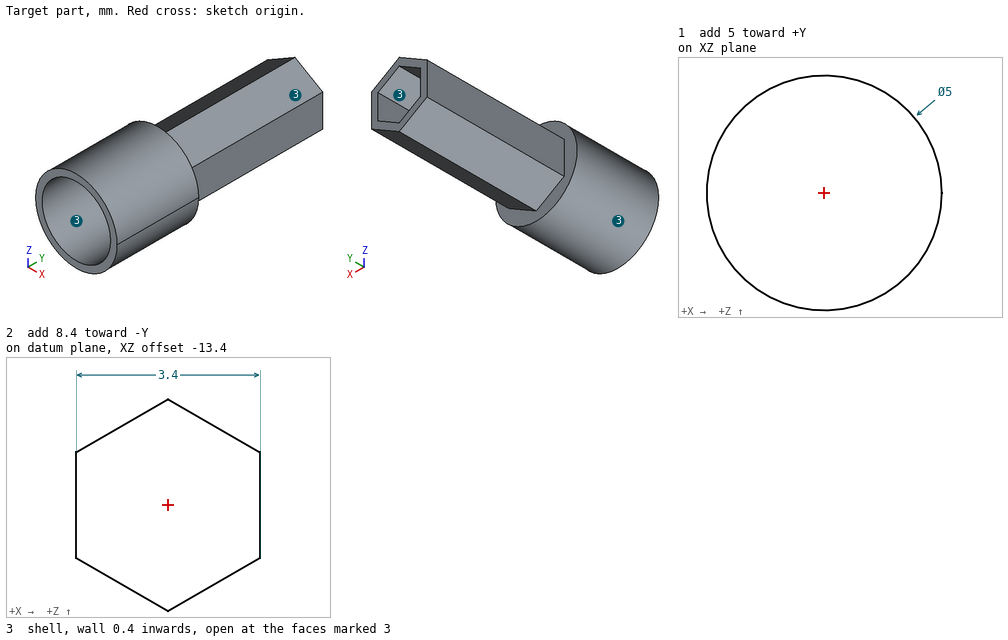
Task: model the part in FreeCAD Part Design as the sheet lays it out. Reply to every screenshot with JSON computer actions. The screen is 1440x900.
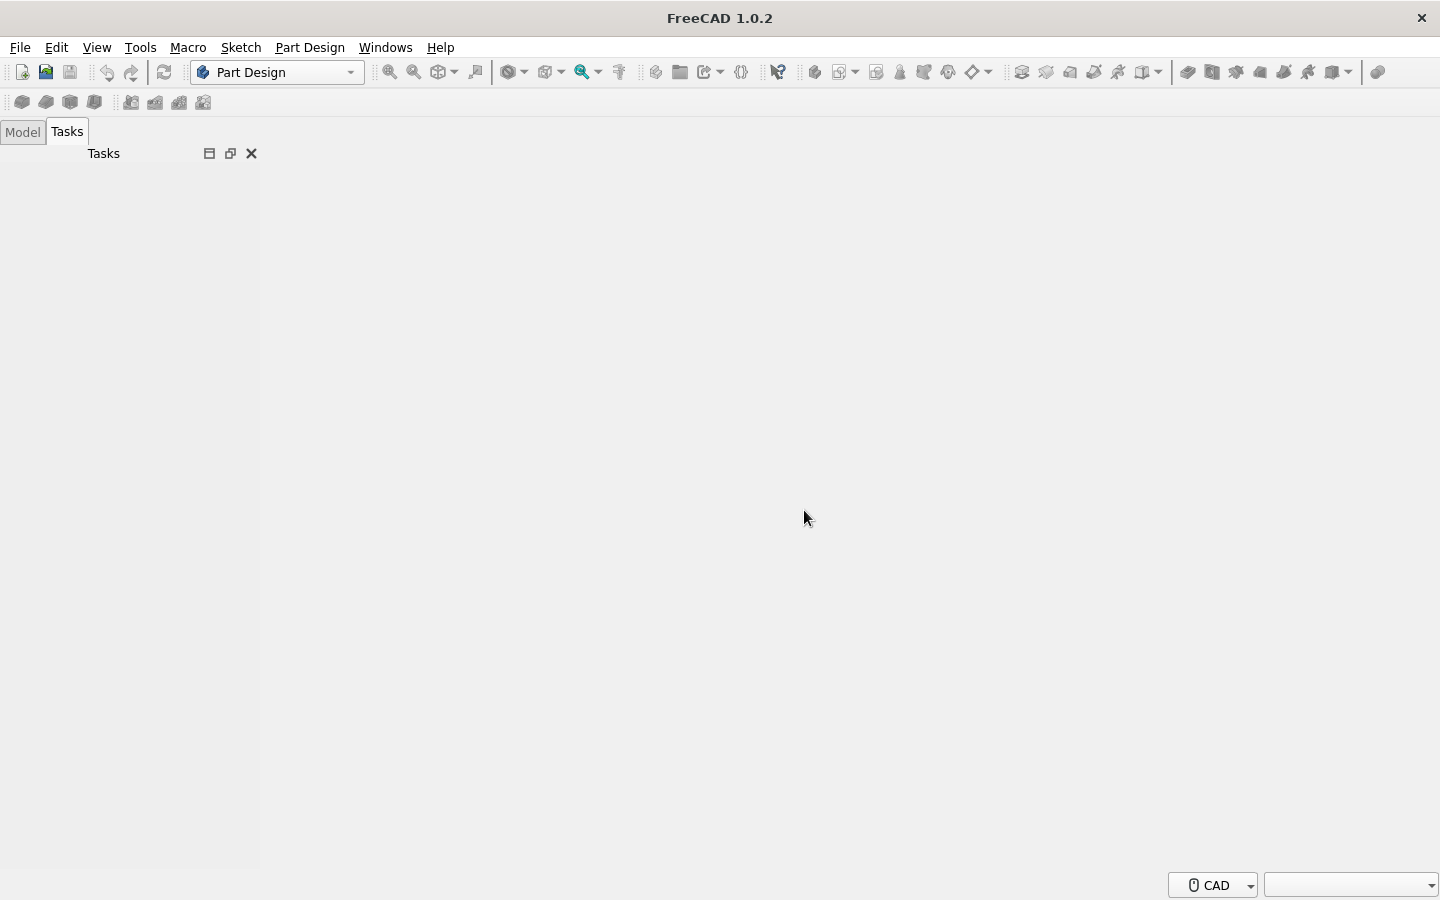
{"action": "left_click", "coordinate": [22, 72]}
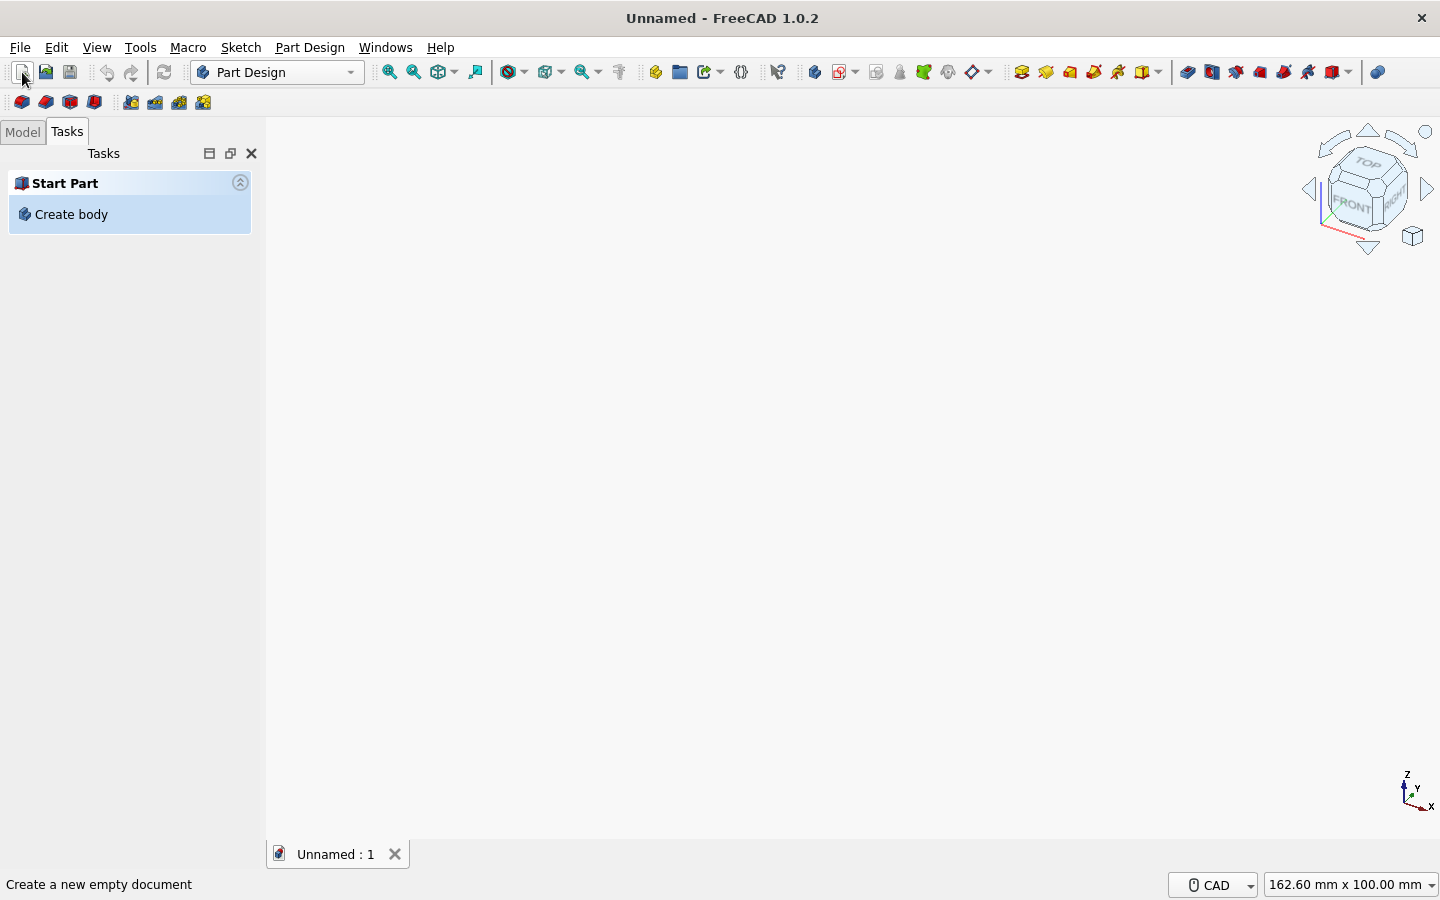
{"action": "left_click", "coordinate": [840, 72]}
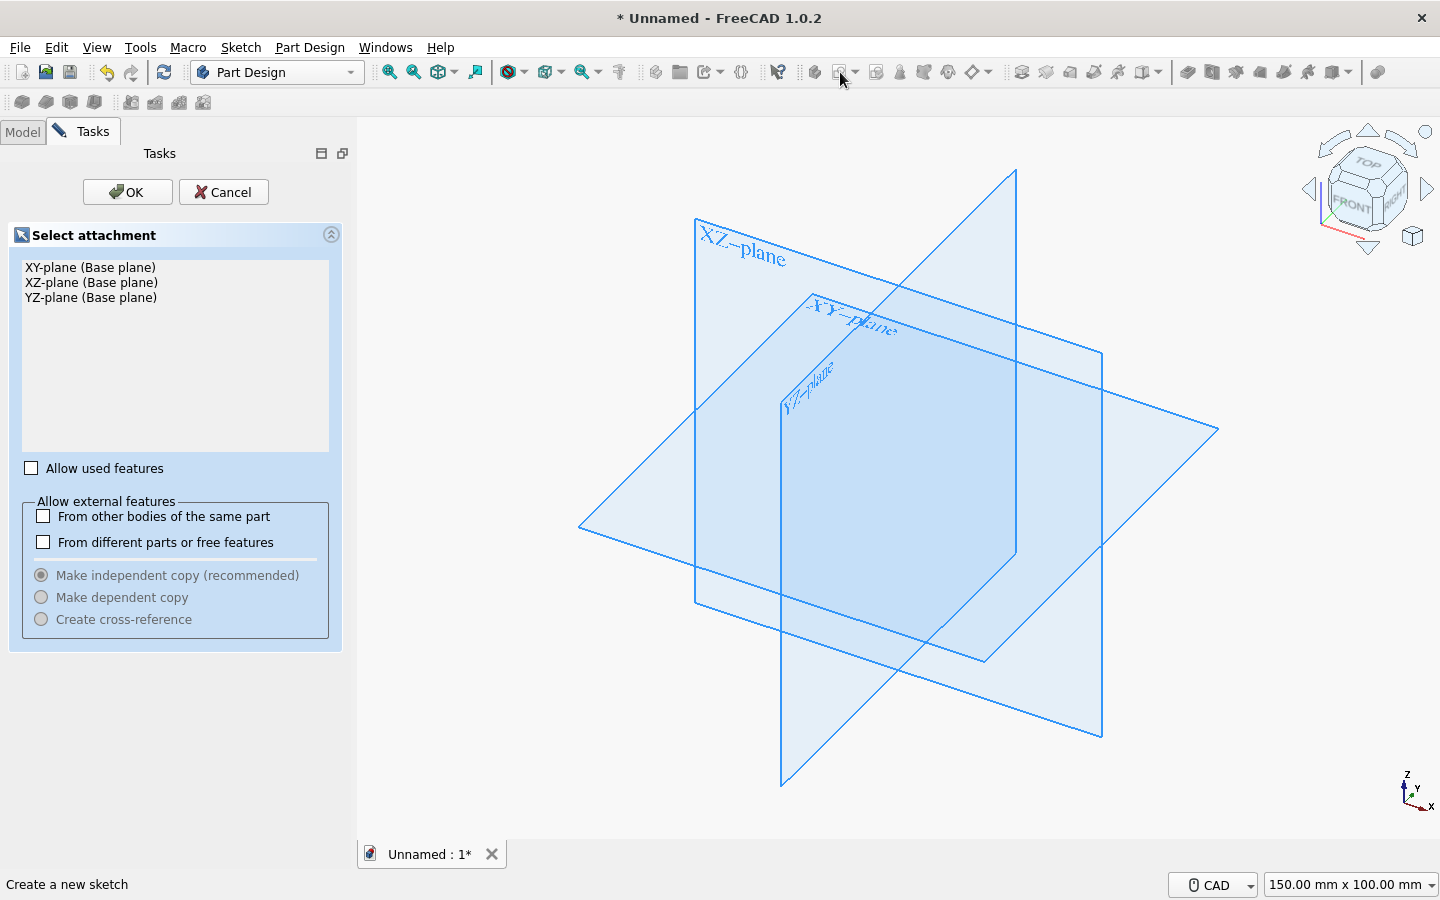
{"action": "left_click", "coordinate": [82, 282]}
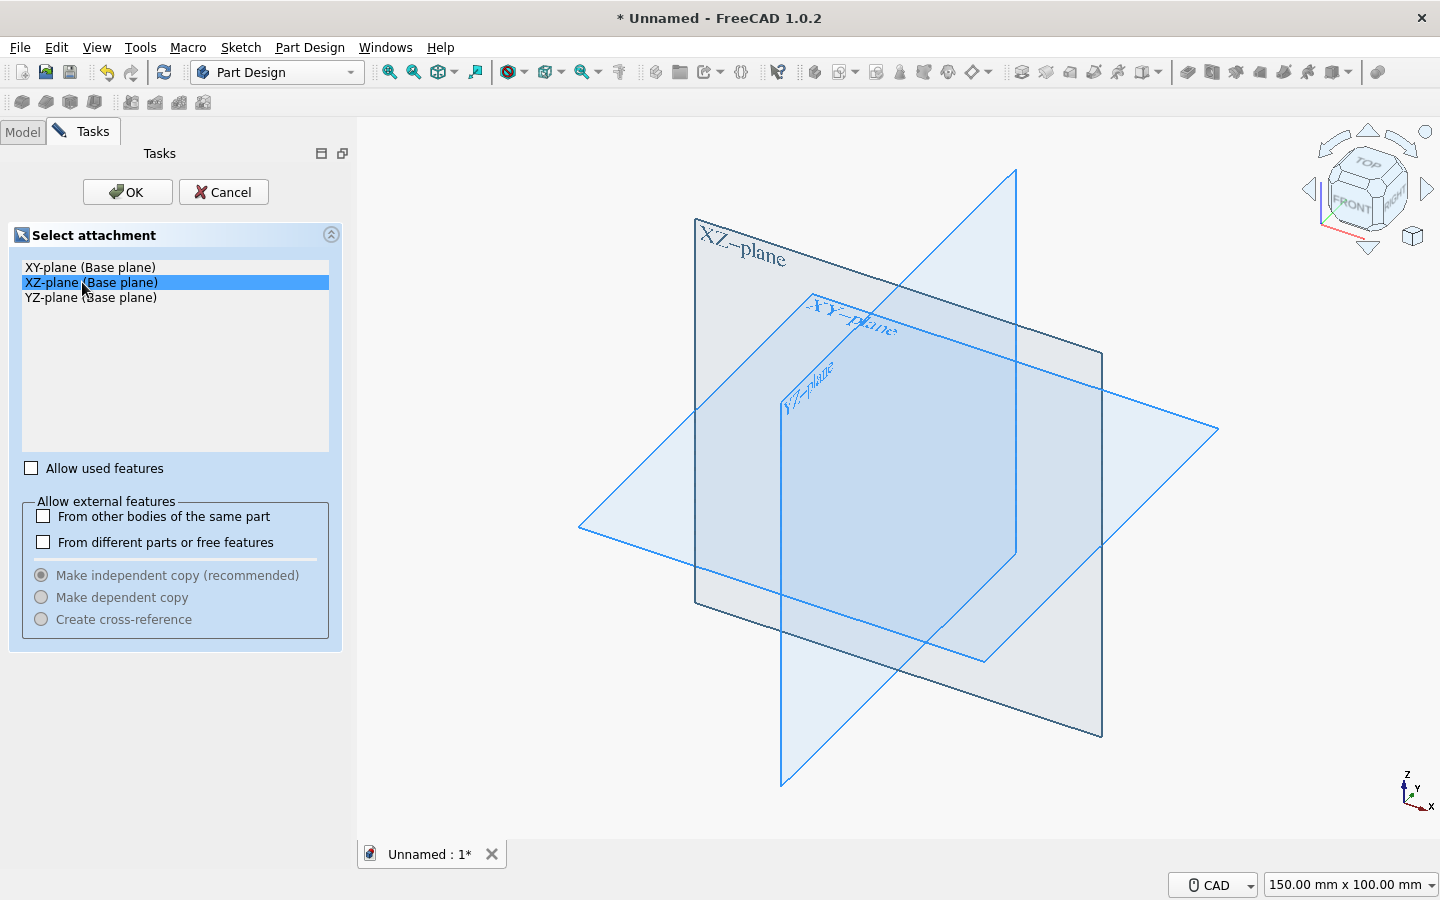
{"action": "left_click", "coordinate": [128, 192]}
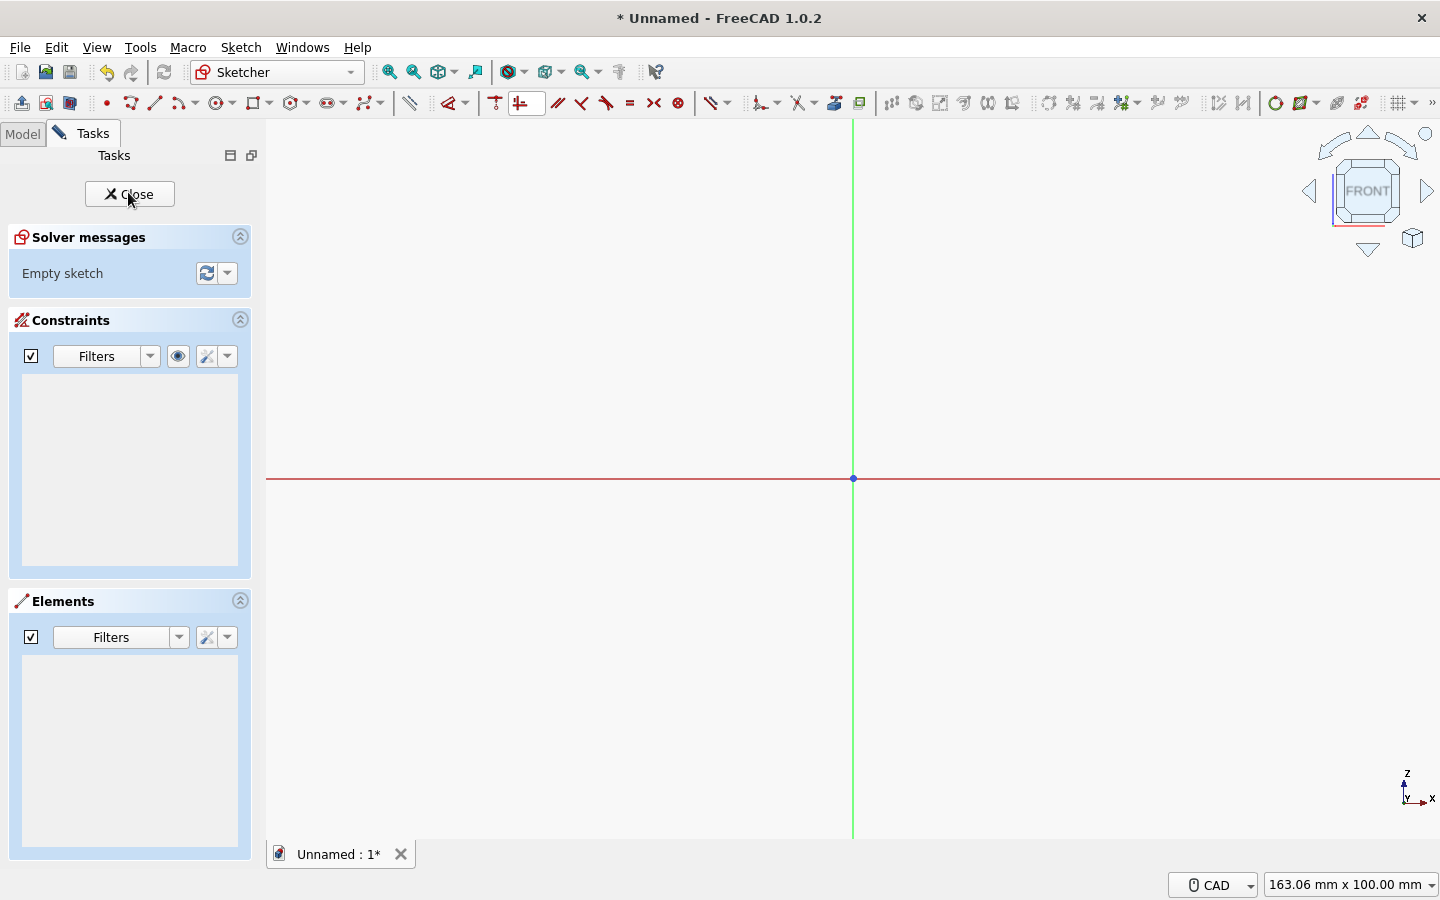
{"action": "scroll", "coordinate": [858, 479], "scroll_direction": "up", "scroll_amount": 13}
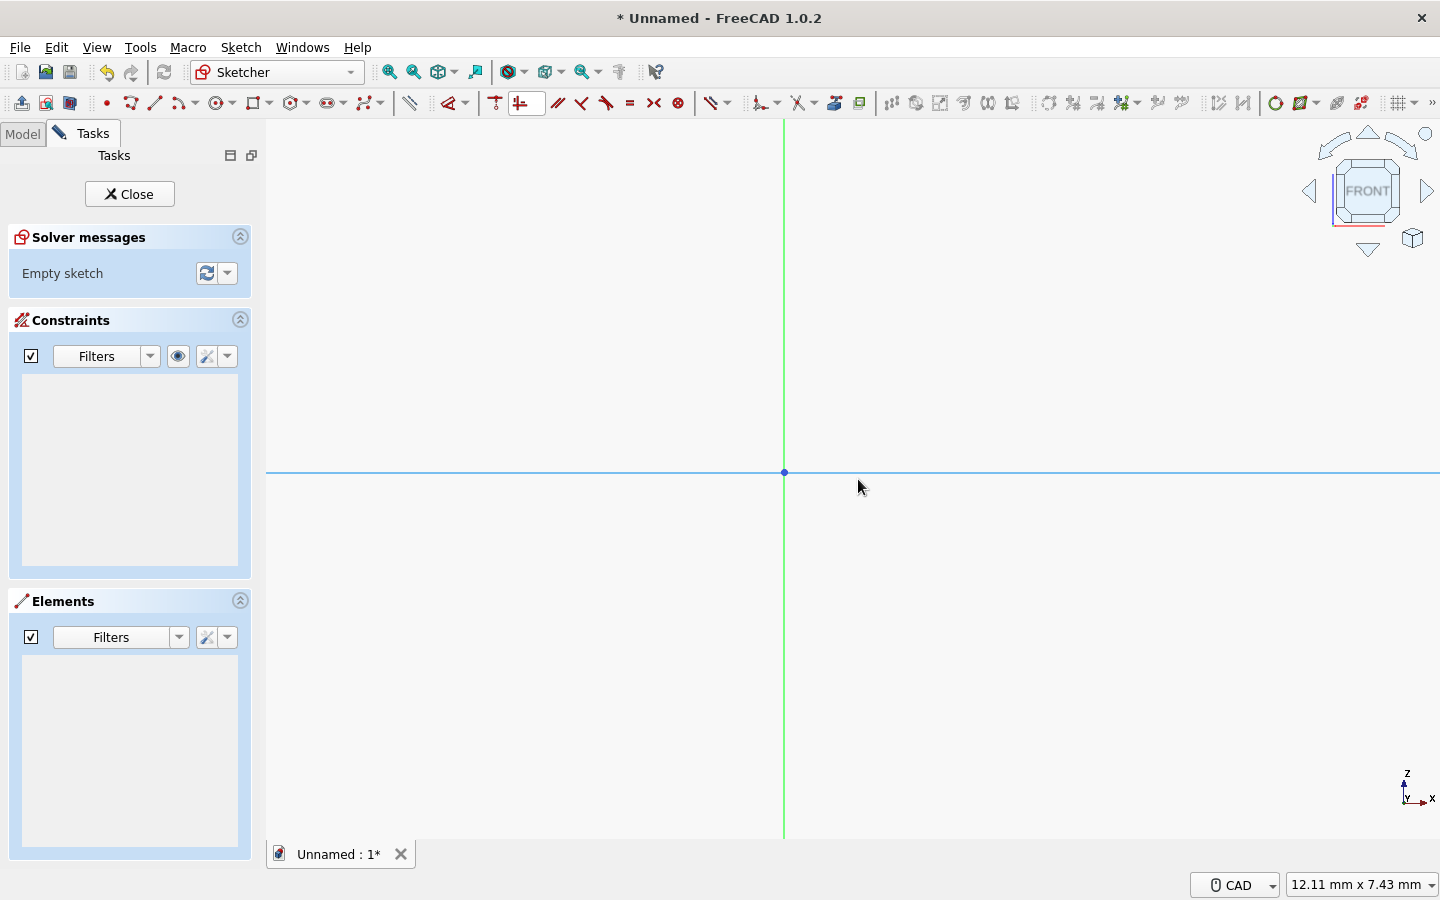
{"action": "left_click", "coordinate": [216, 104]}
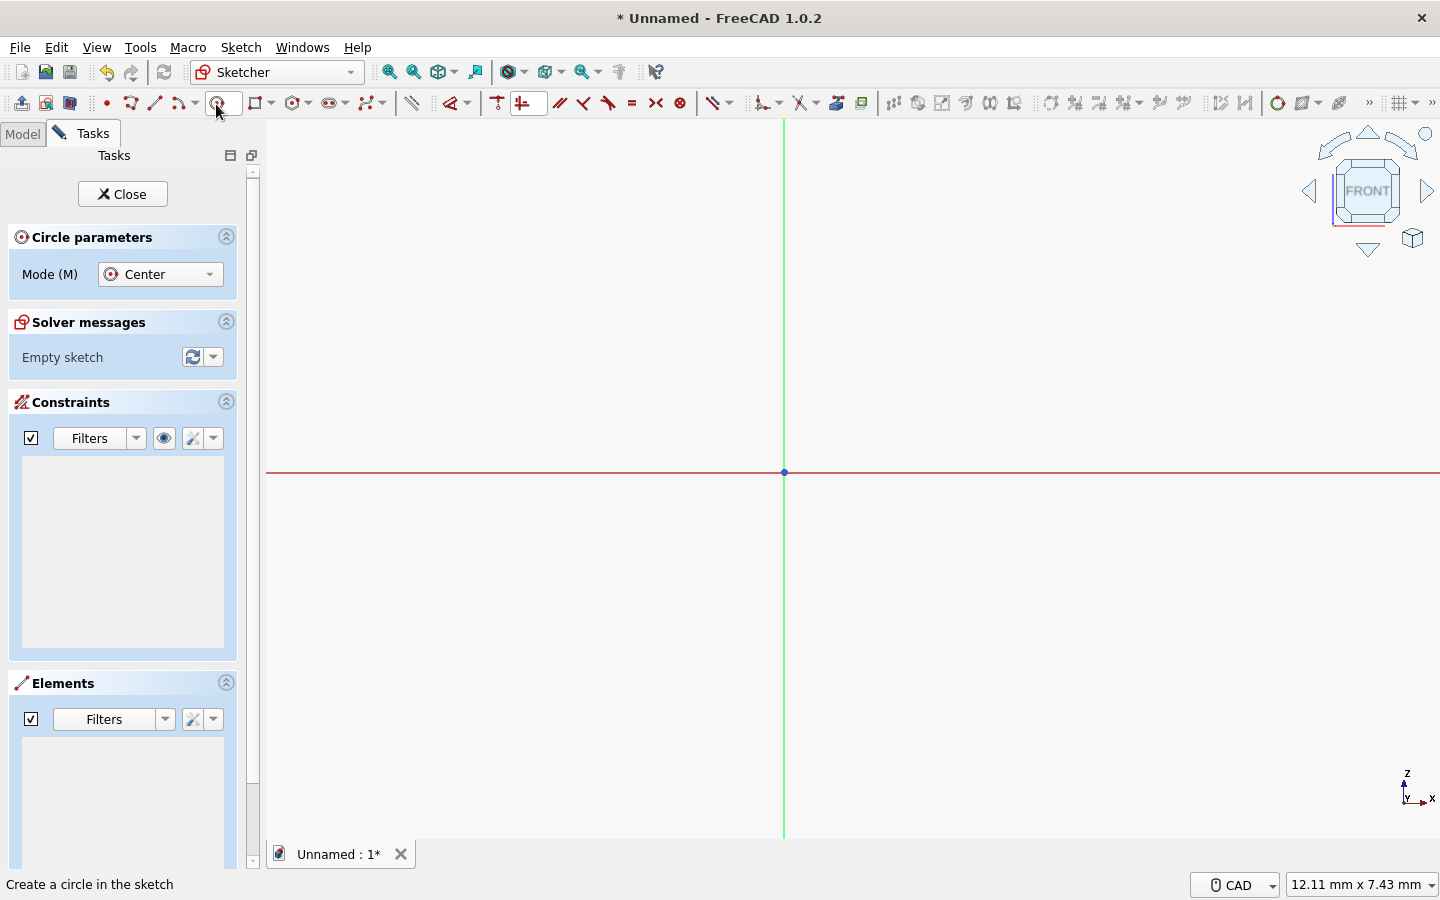
{"action": "left_click", "coordinate": [784, 473]}
{"action": "mouse_move", "coordinate": [956, 301]}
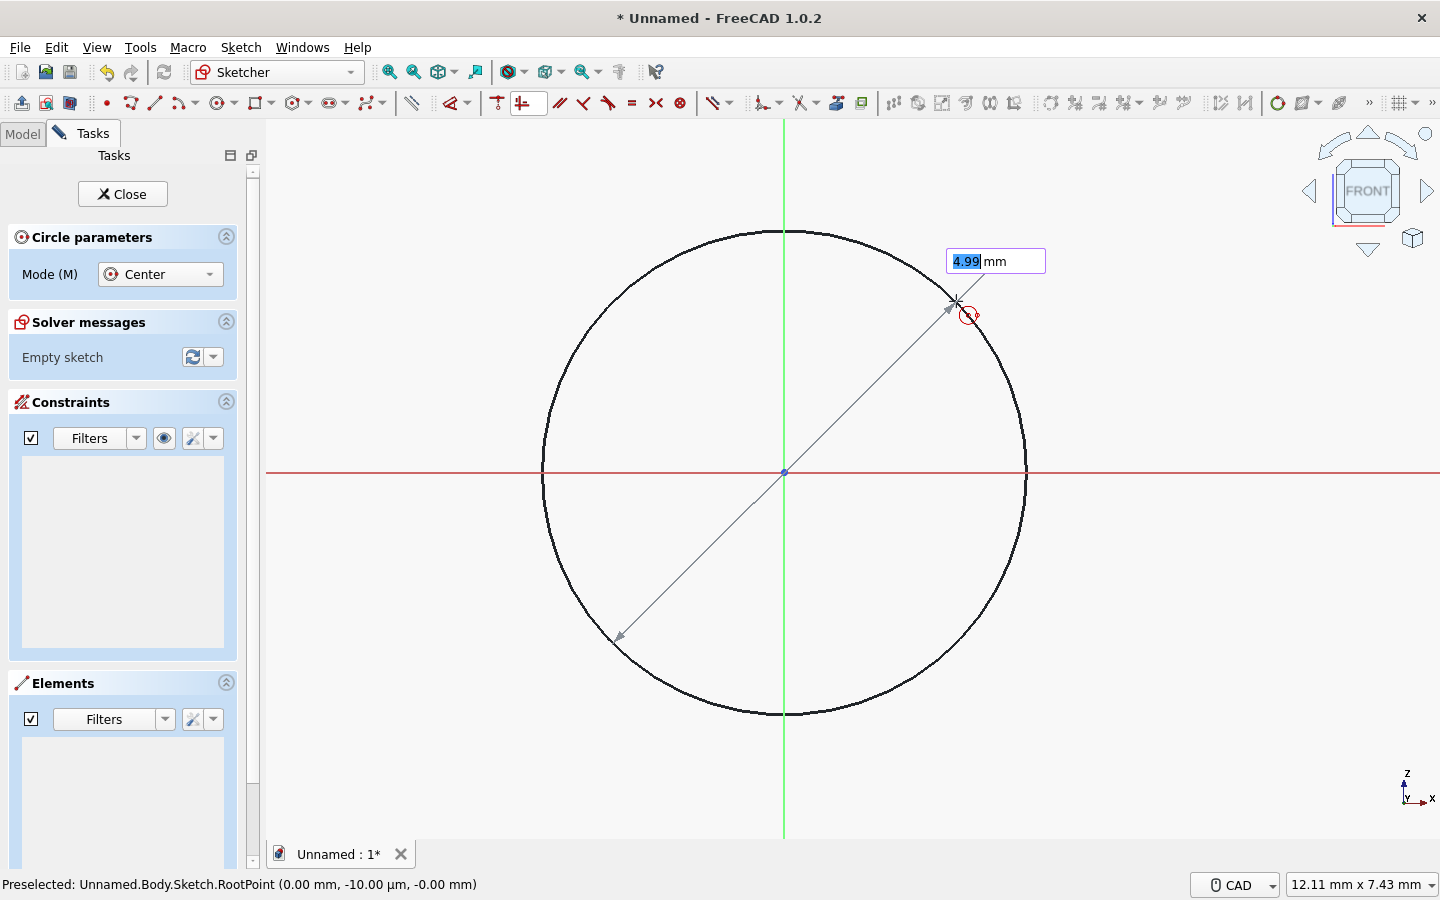
{"action": "type", "text": "5"}
{"action": "key", "text": "Return"}
{"action": "key", "text": "Escape"}